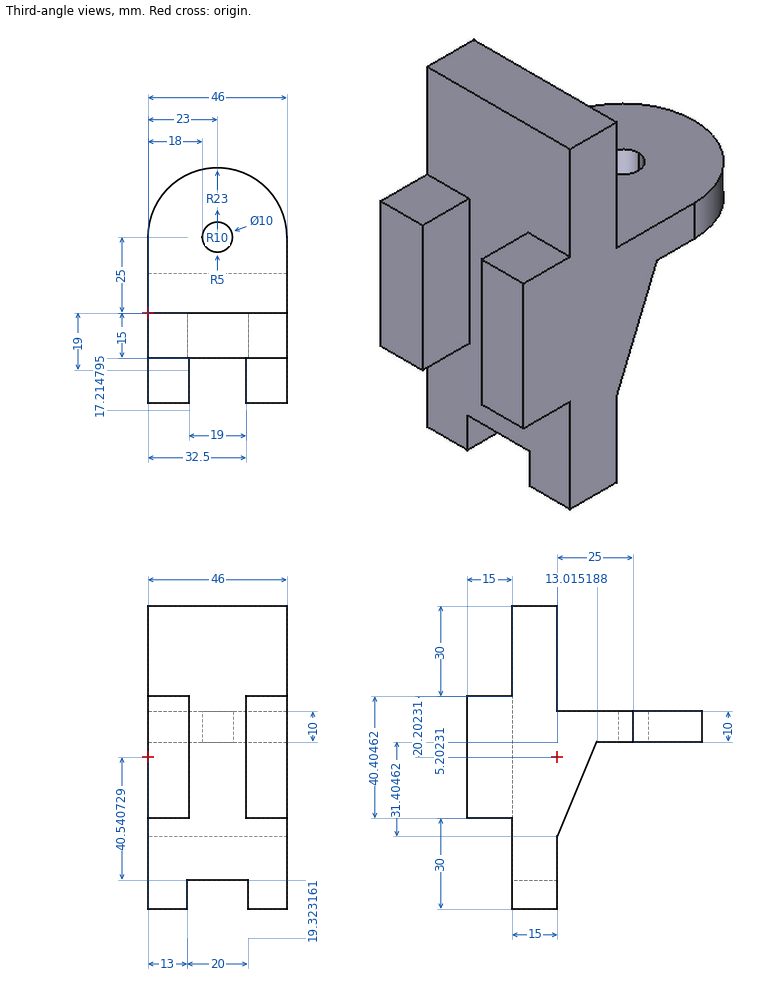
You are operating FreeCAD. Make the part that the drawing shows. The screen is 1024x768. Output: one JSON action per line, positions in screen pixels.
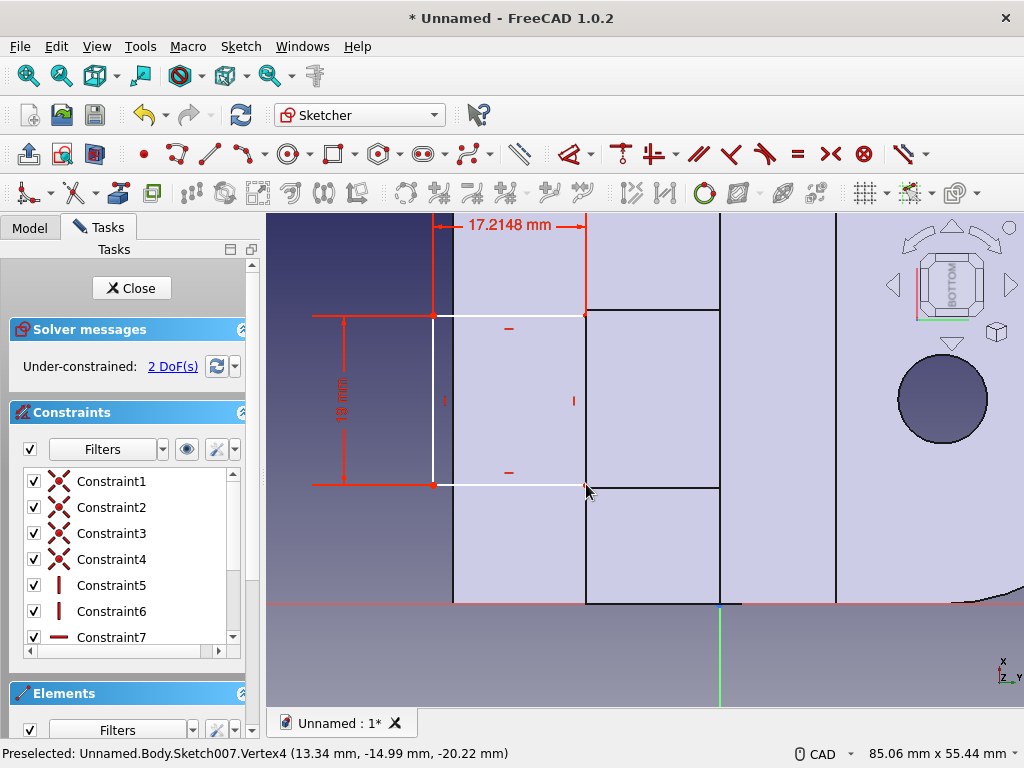
{"action": "key", "text": "d"}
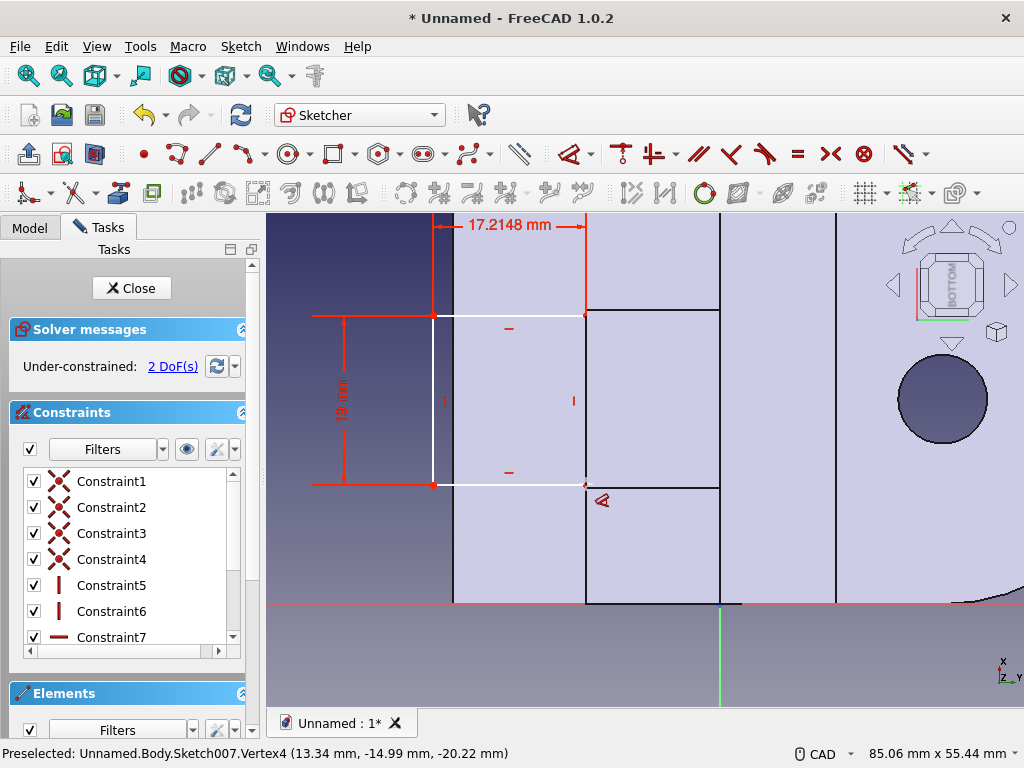
{"action": "left_click", "coordinate": [586, 485]}
{"action": "left_click", "coordinate": [653, 638]}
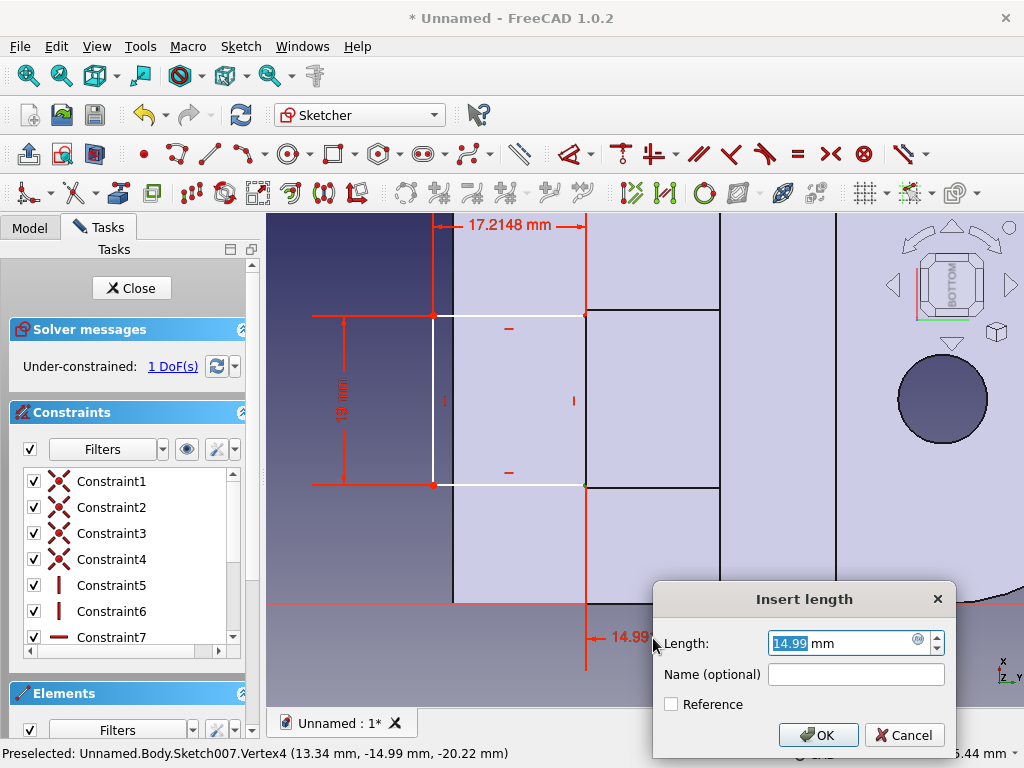
{"action": "type", "text": "15"}
{"action": "key", "text": "Return"}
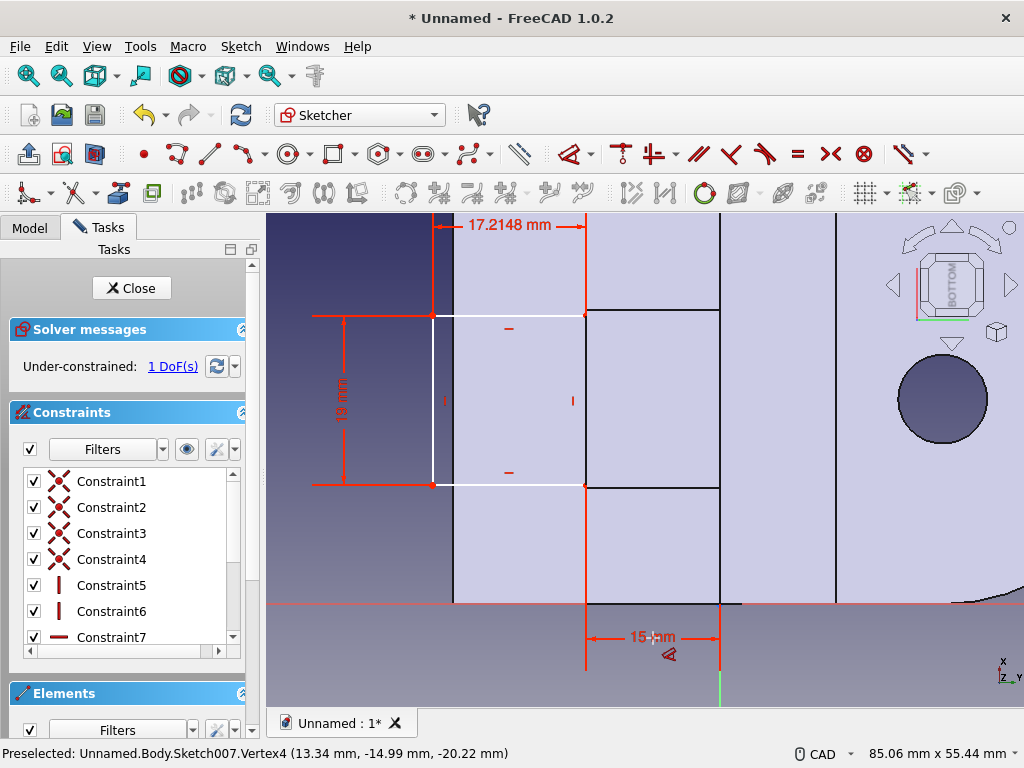
{"action": "left_click", "coordinate": [433, 316]}
{"action": "left_click", "coordinate": [754, 460]}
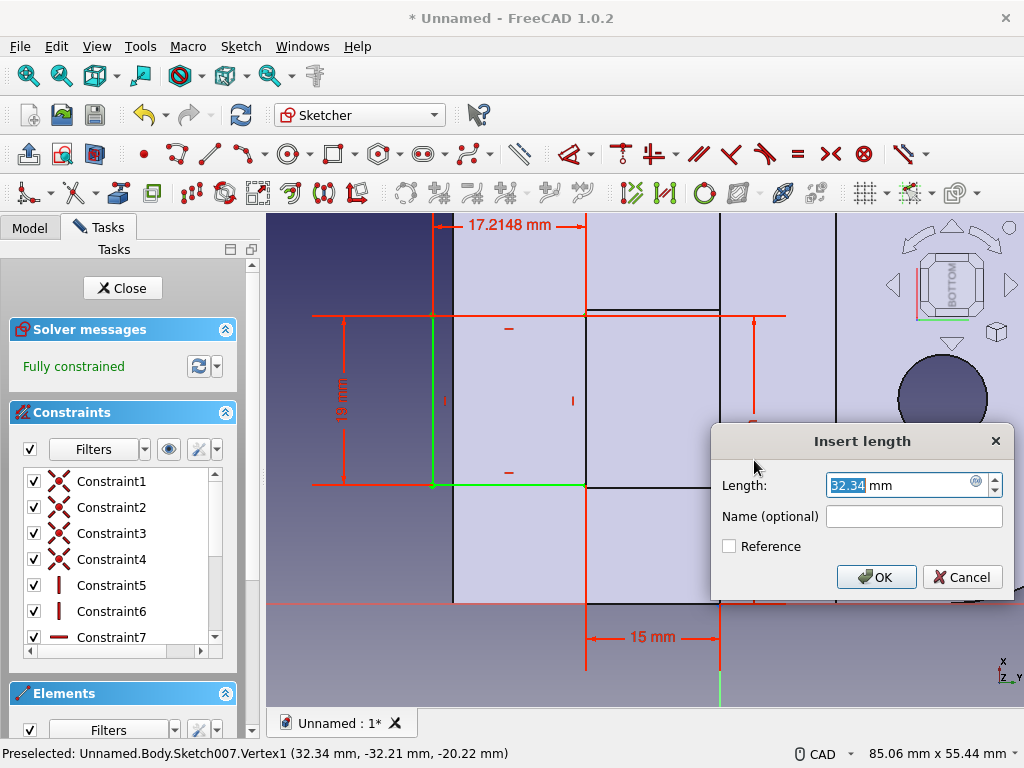
{"action": "type", "text": "32.5"}
{"action": "key", "text": "Return"}
{"action": "key", "text": "Escape"}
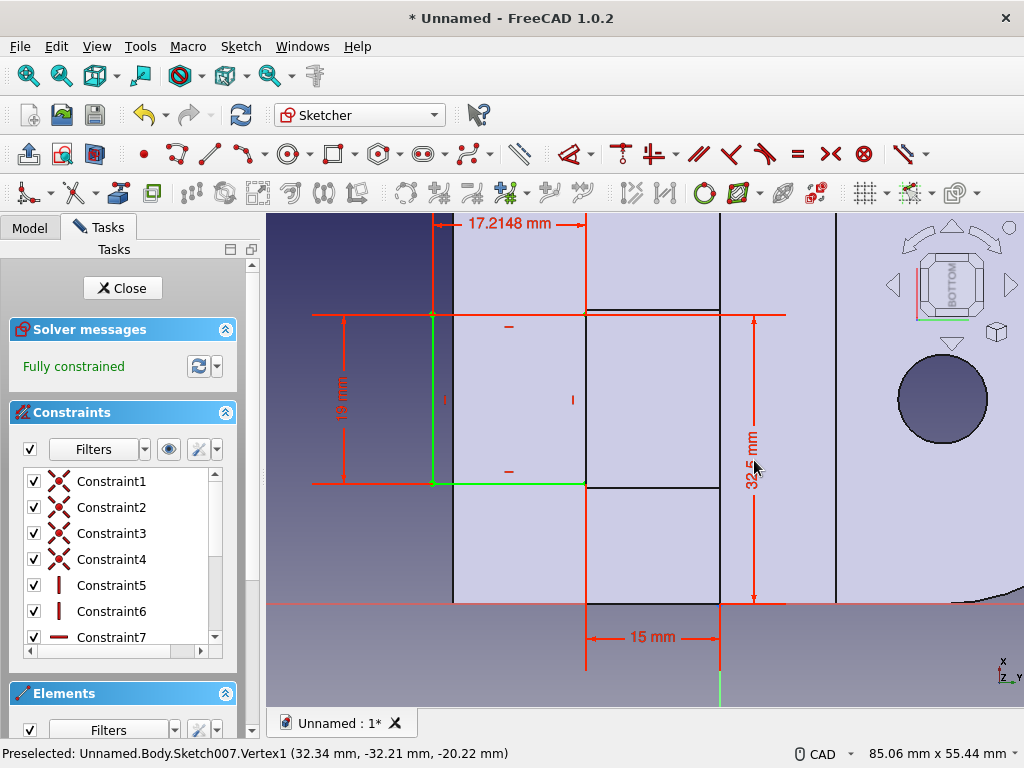
{"action": "left_click", "coordinate": [123, 288]}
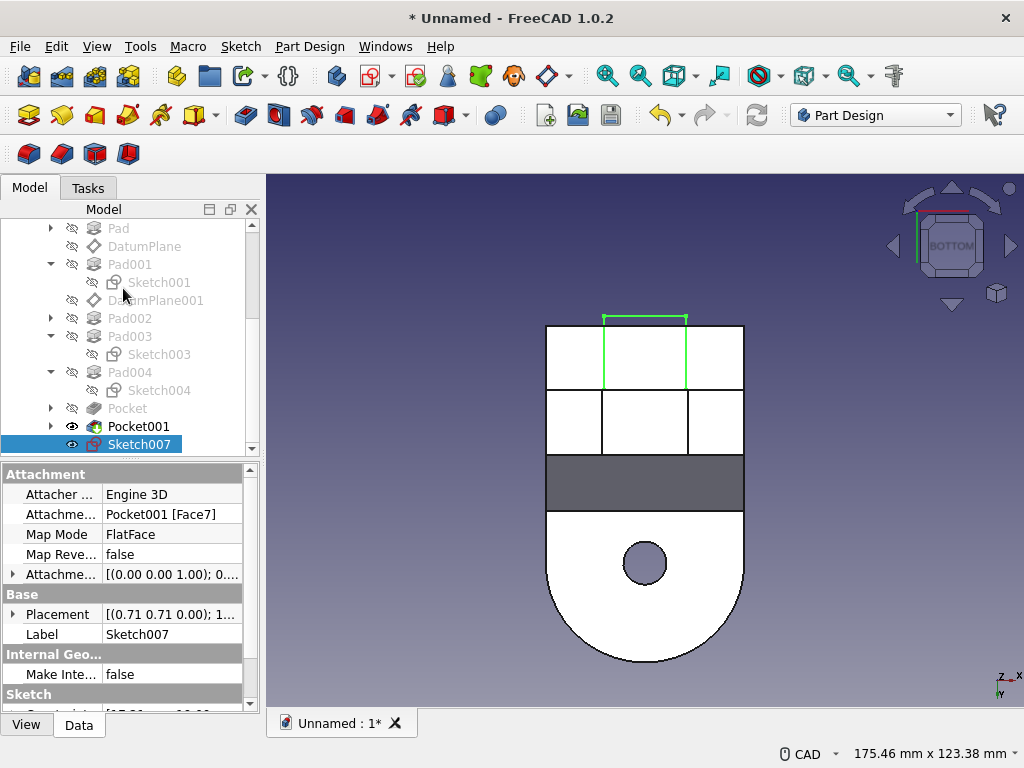
{"action": "left_click", "coordinate": [246, 116]}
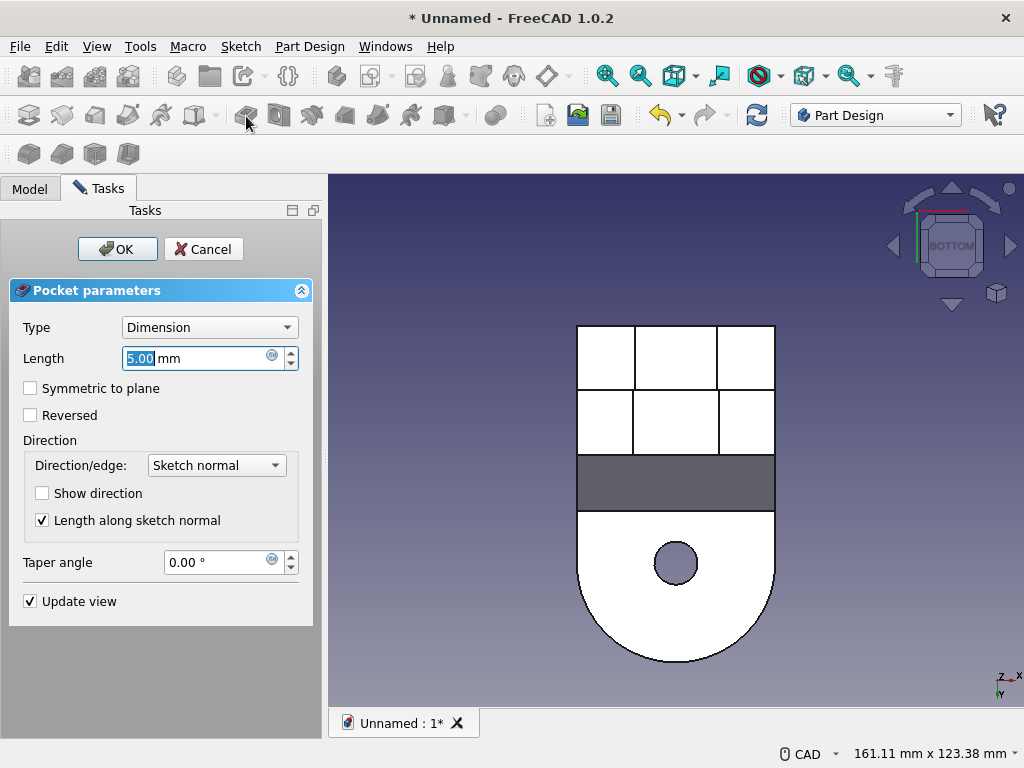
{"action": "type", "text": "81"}
{"action": "key", "text": "Tab"}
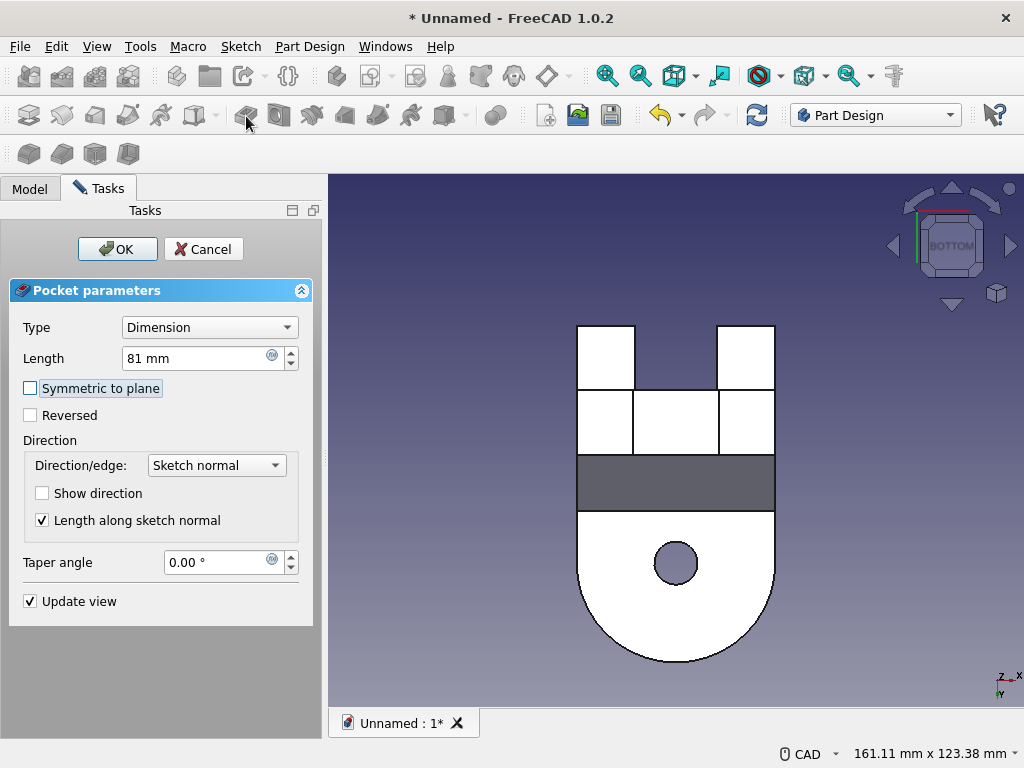
{"action": "left_click", "coordinate": [118, 249]}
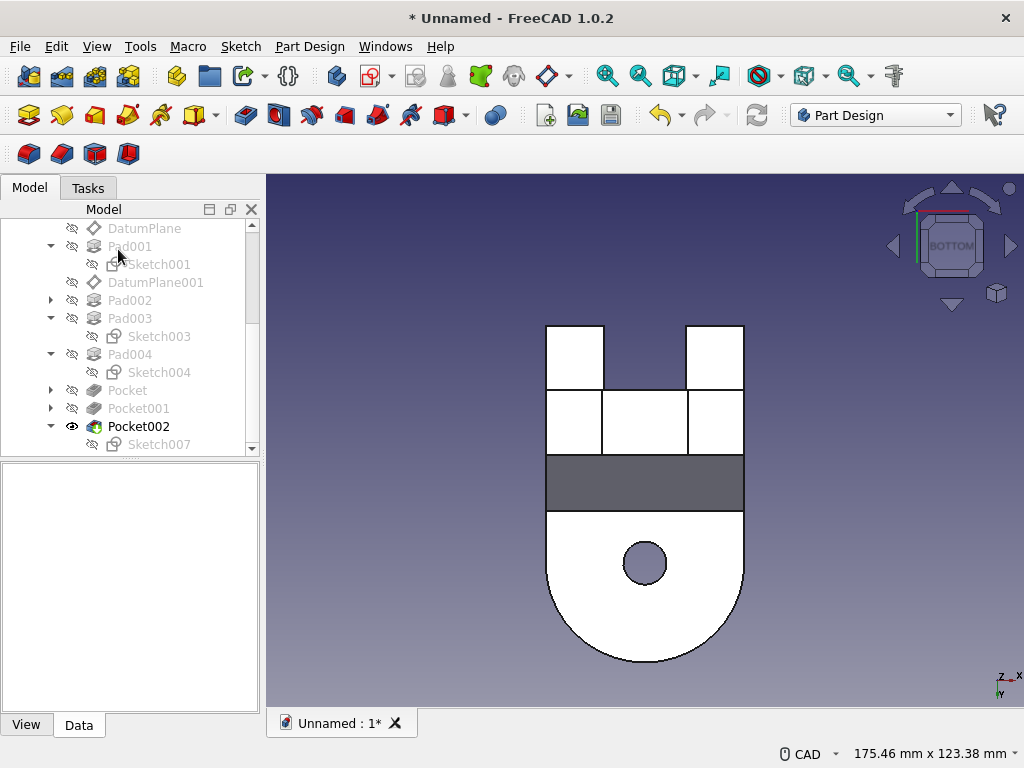
{"action": "key", "text": "0"}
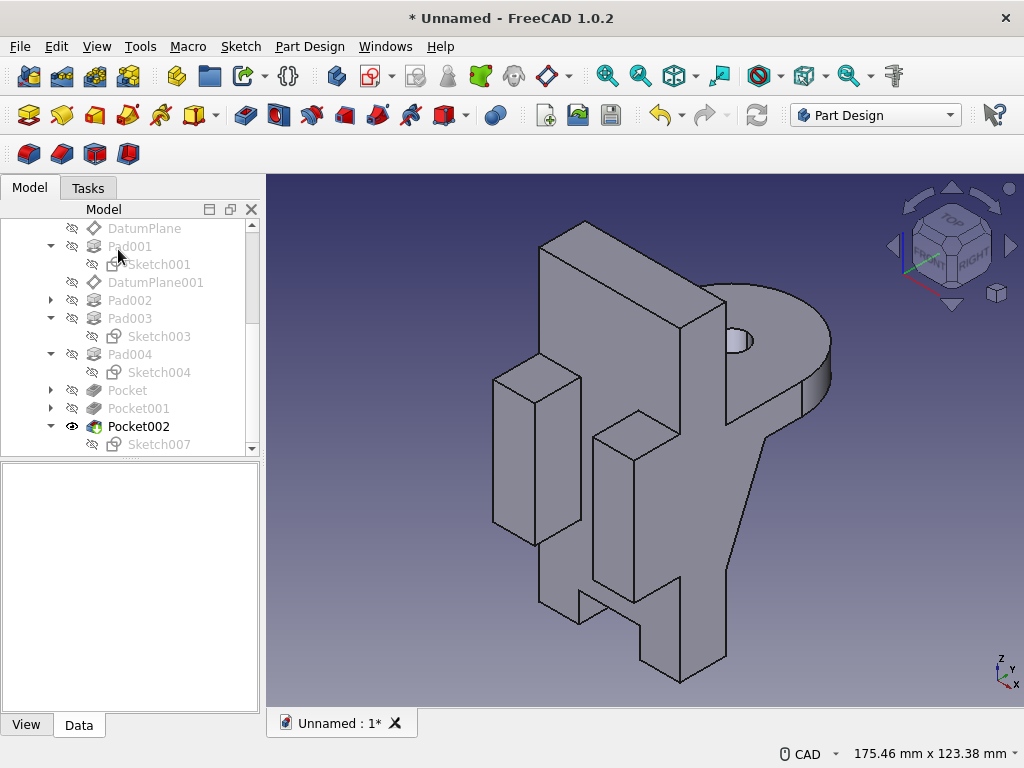
{"action": "key", "text": "v f"}